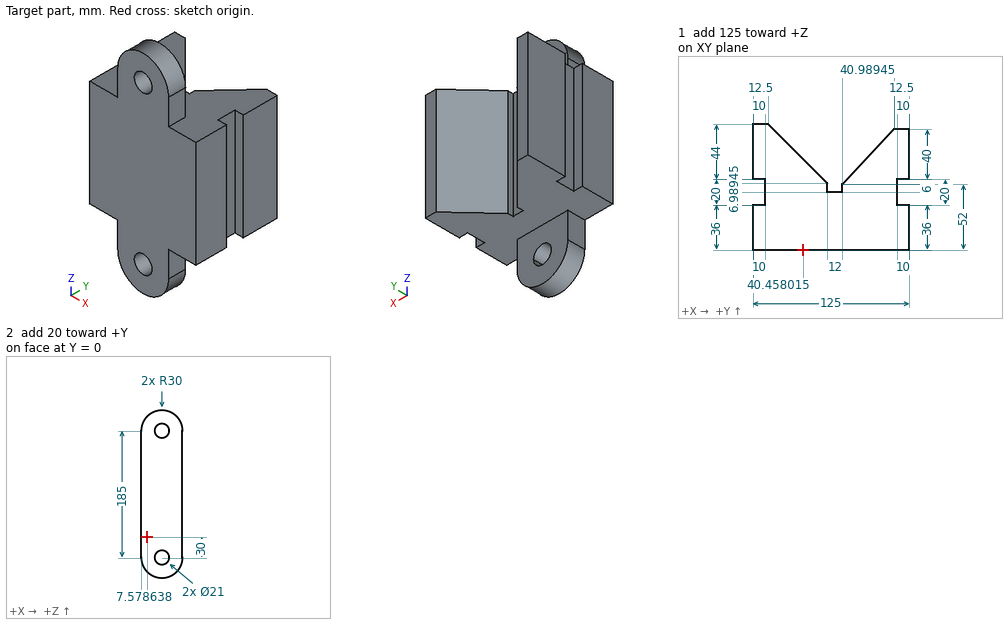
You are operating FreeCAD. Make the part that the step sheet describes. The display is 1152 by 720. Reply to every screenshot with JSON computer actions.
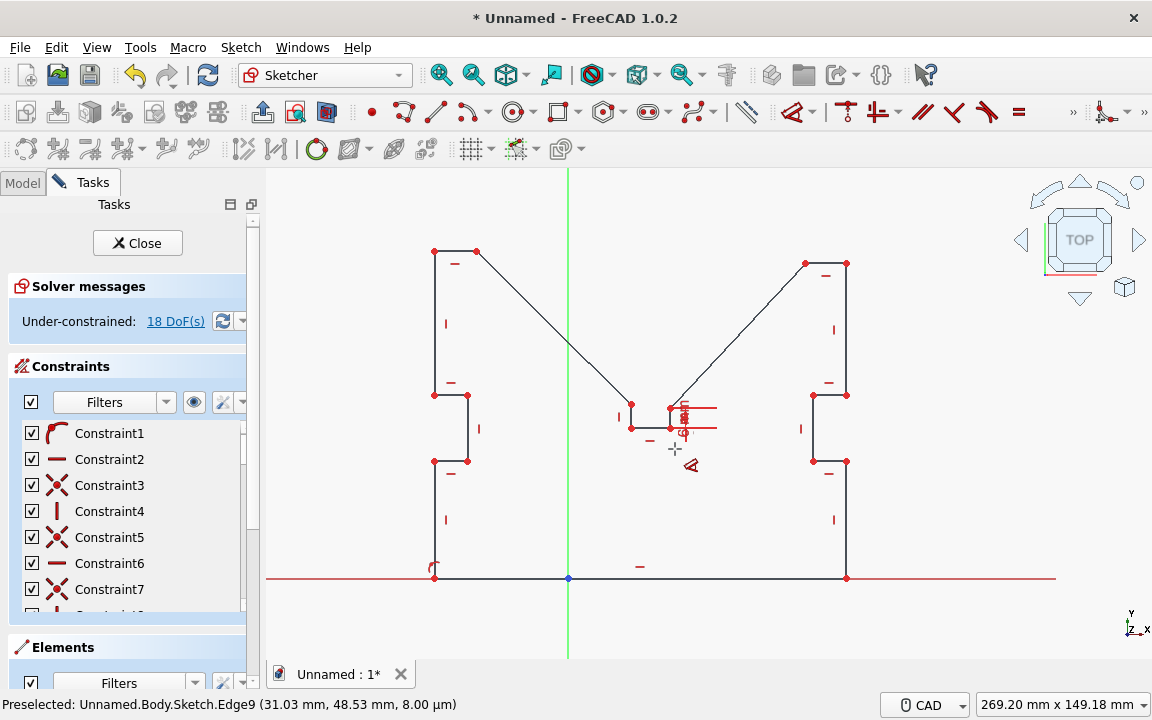
{"action": "left_click", "coordinate": [846, 543]}
{"action": "left_click", "coordinate": [880, 520]}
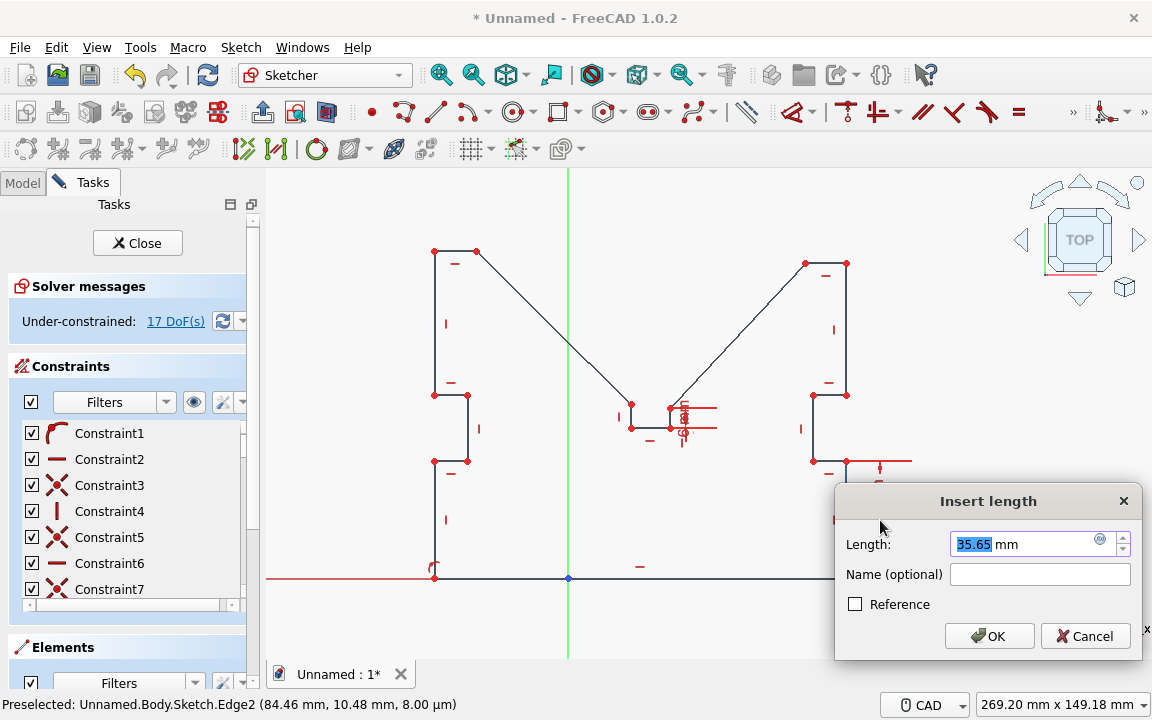
{"action": "type", "text": "36"}
{"action": "key", "text": "Return"}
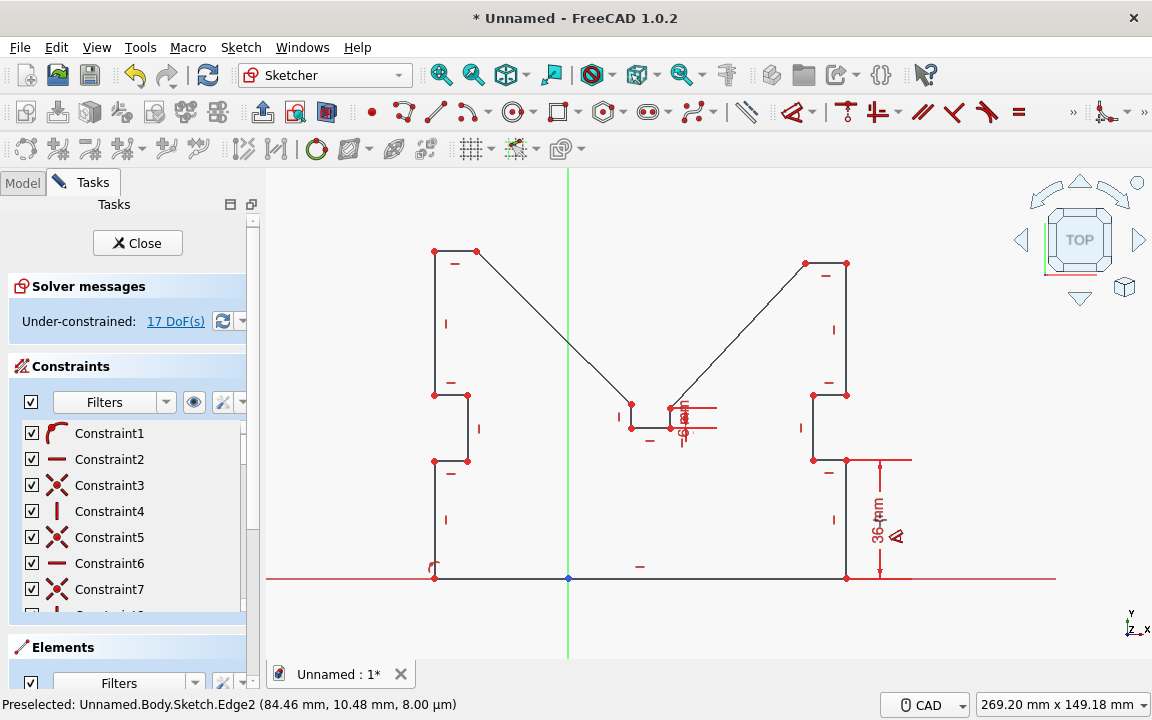
{"action": "scroll", "coordinate": [836, 460], "scroll_direction": "up", "scroll_amount": 2}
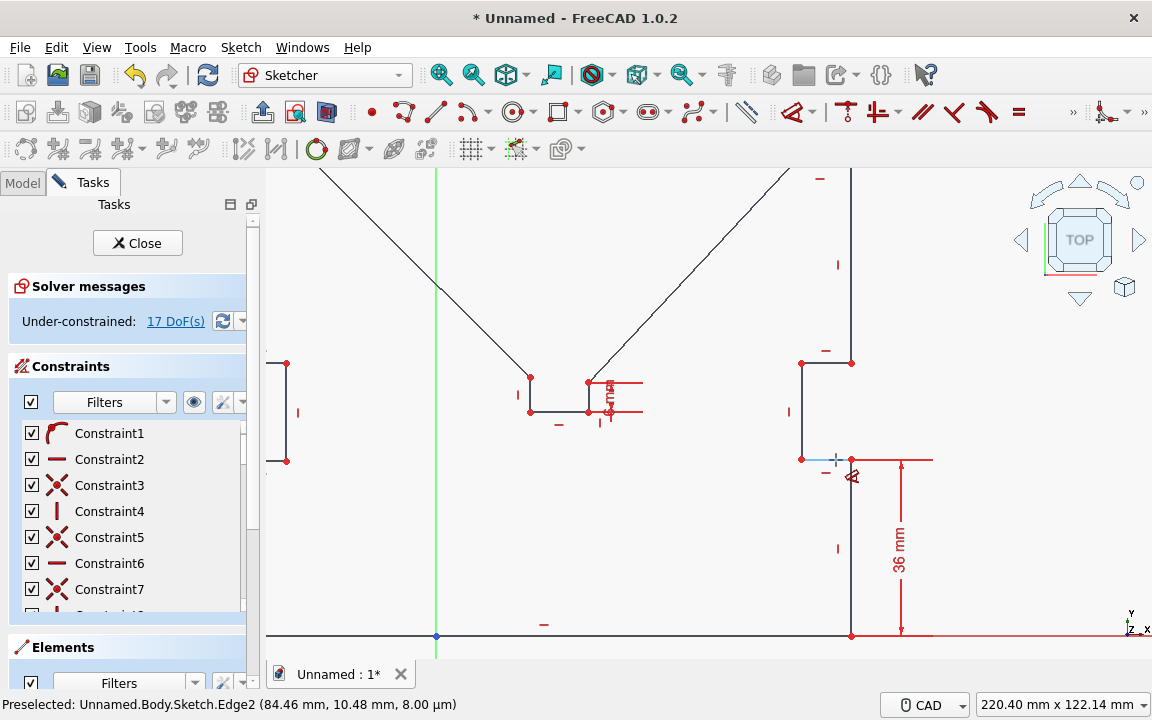
{"action": "left_click", "coordinate": [836, 460]}
{"action": "left_click", "coordinate": [826, 494]}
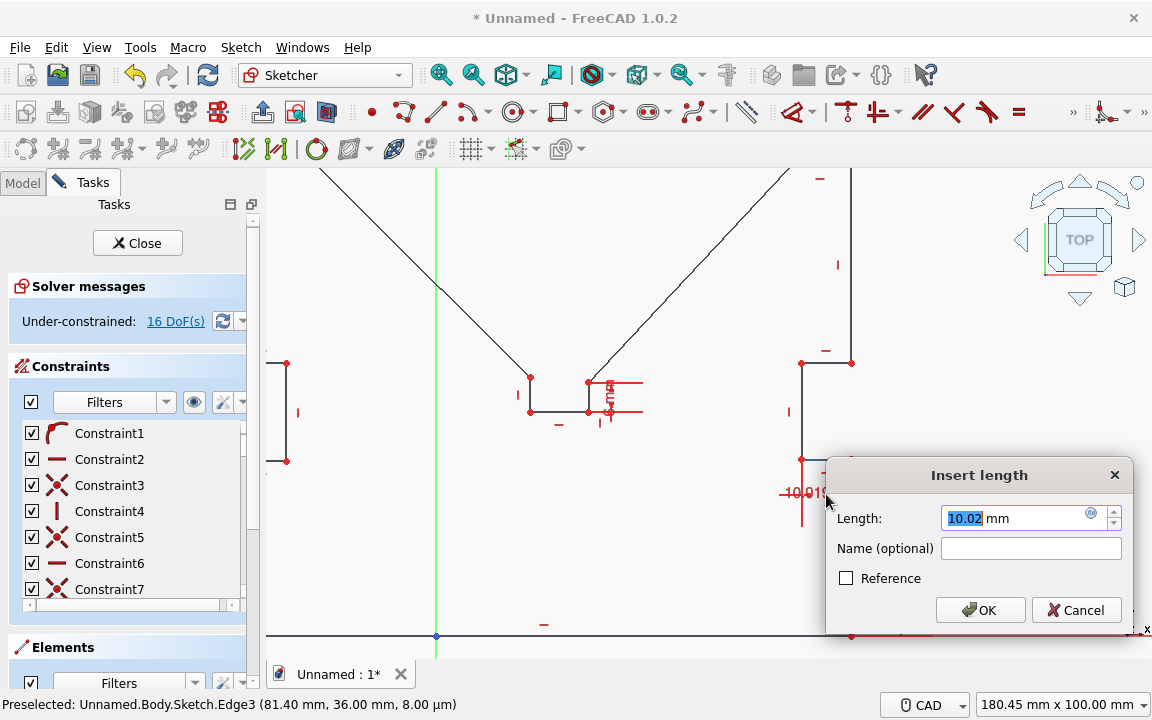
{"action": "type", "text": "10"}
{"action": "key", "text": "Return"}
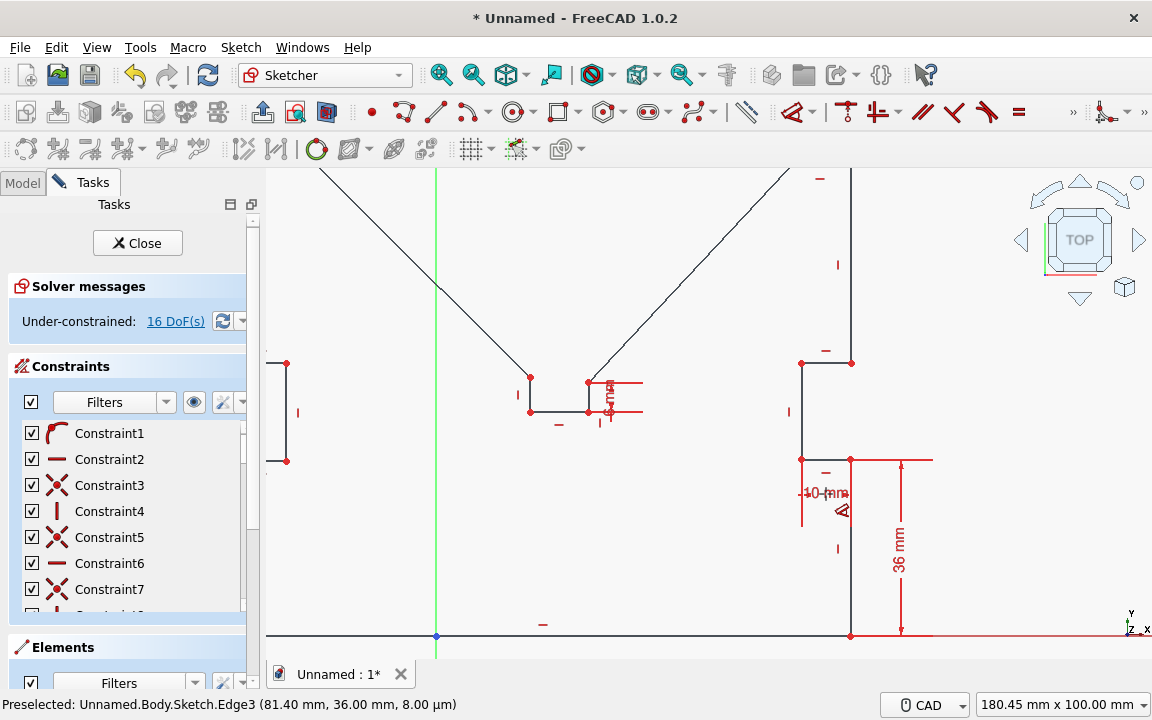
{"action": "left_click", "coordinate": [802, 431]}
{"action": "left_click", "coordinate": [836, 411]}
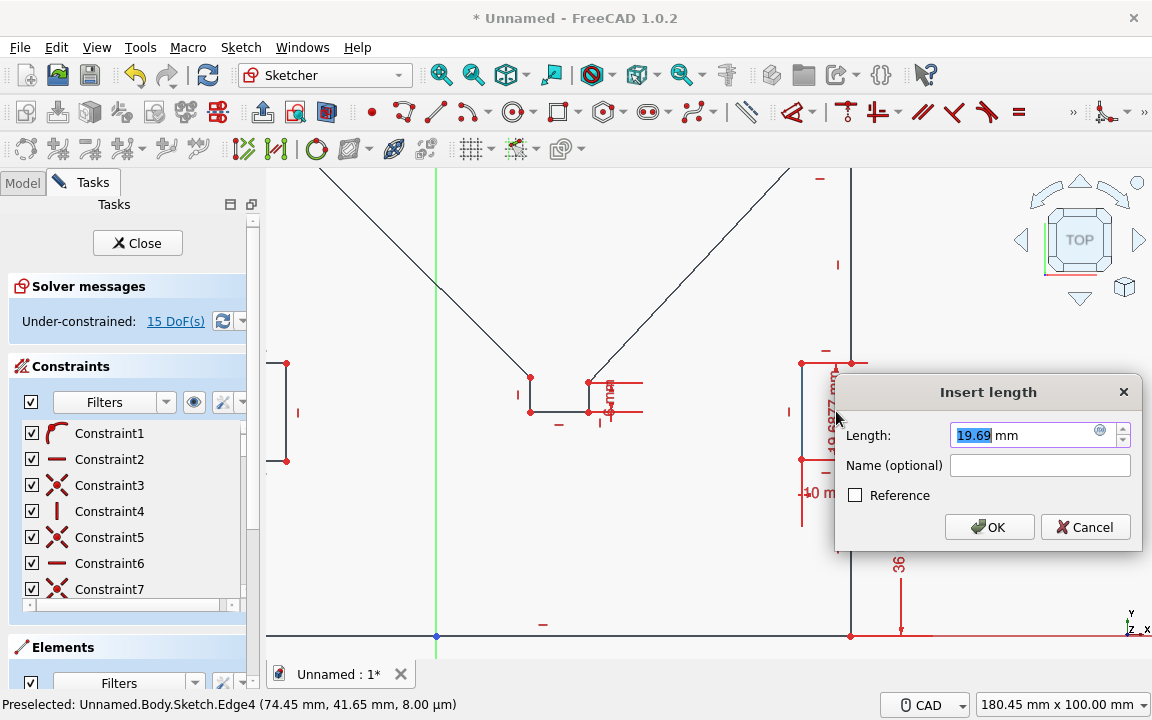
{"action": "type", "text": "20"}
{"action": "key", "text": "Return"}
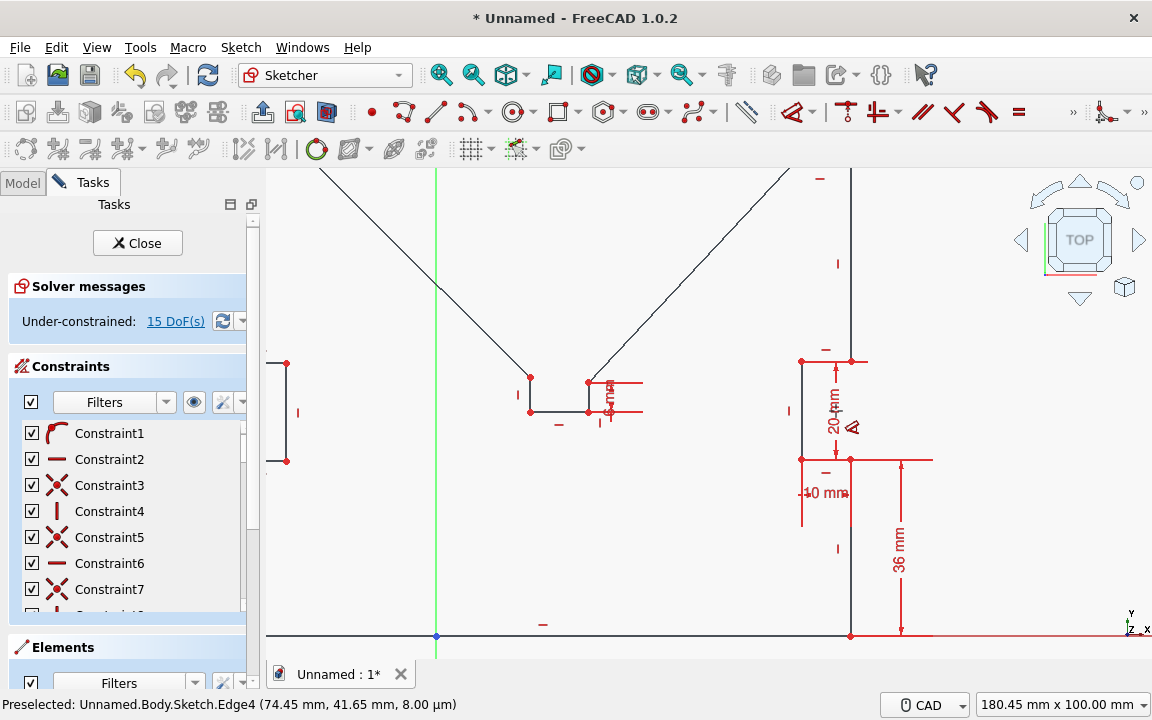
{"action": "left_click", "coordinate": [817, 362]}
{"action": "left_click", "coordinate": [826, 328]}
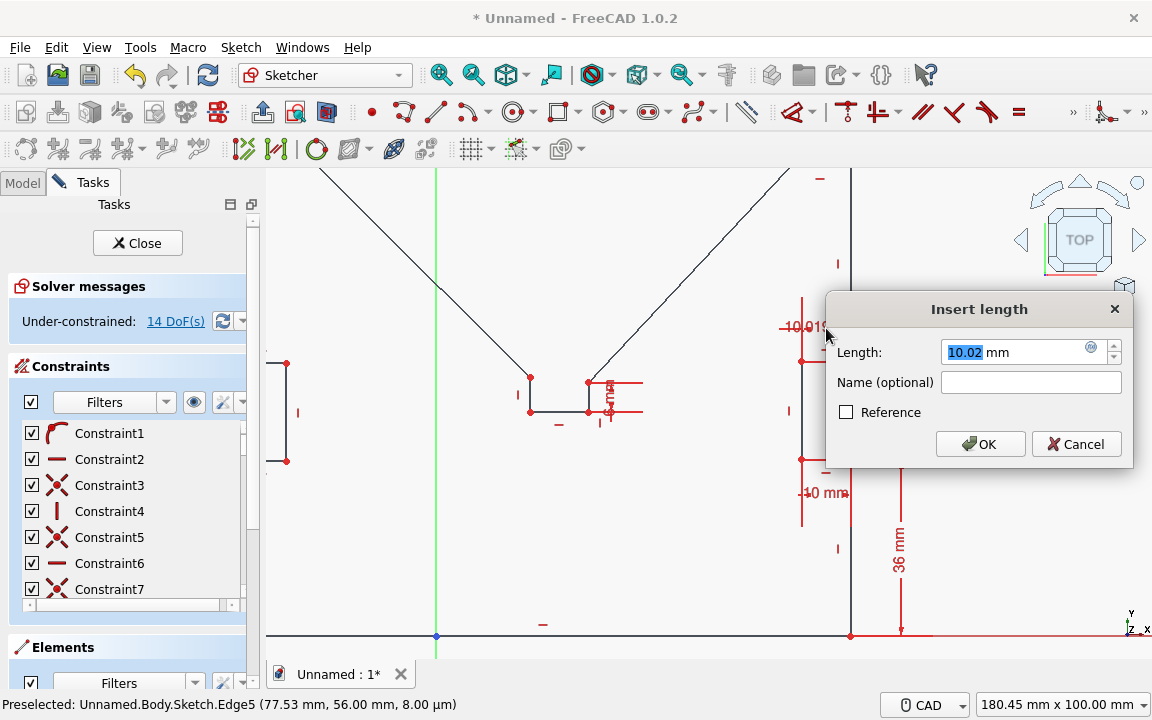
{"action": "type", "text": "10"}
{"action": "key", "text": "Return"}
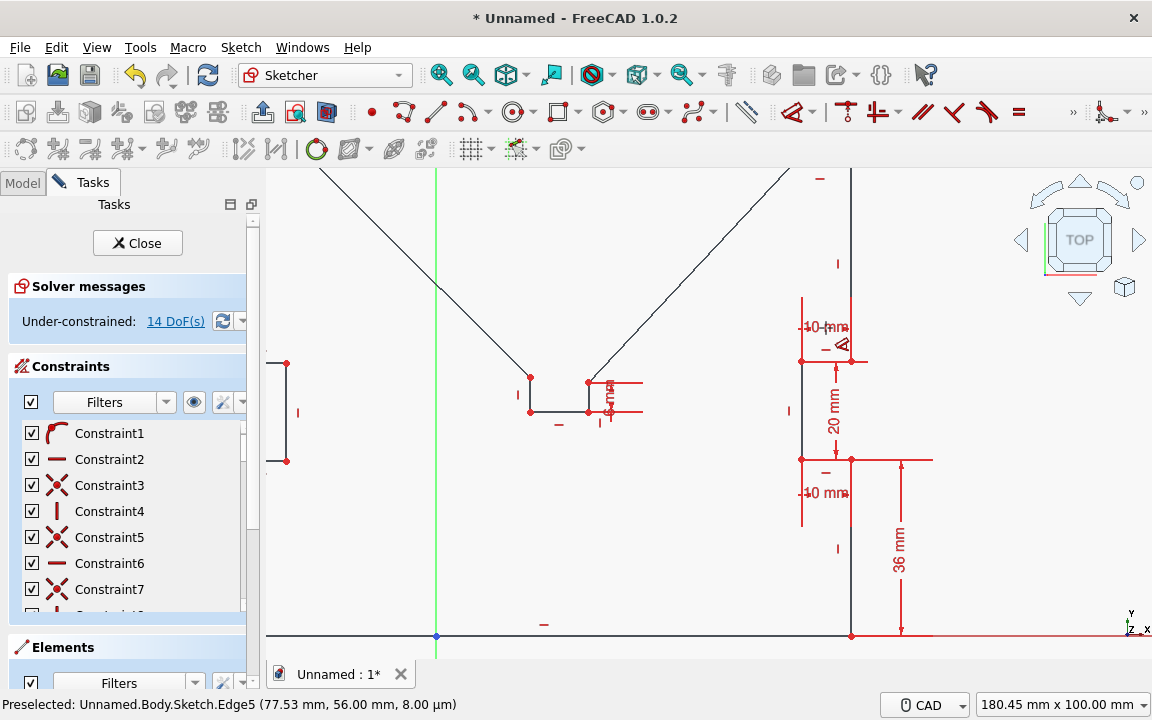
{"action": "left_click", "coordinate": [851, 303]}
{"action": "left_click", "coordinate": [885, 279]}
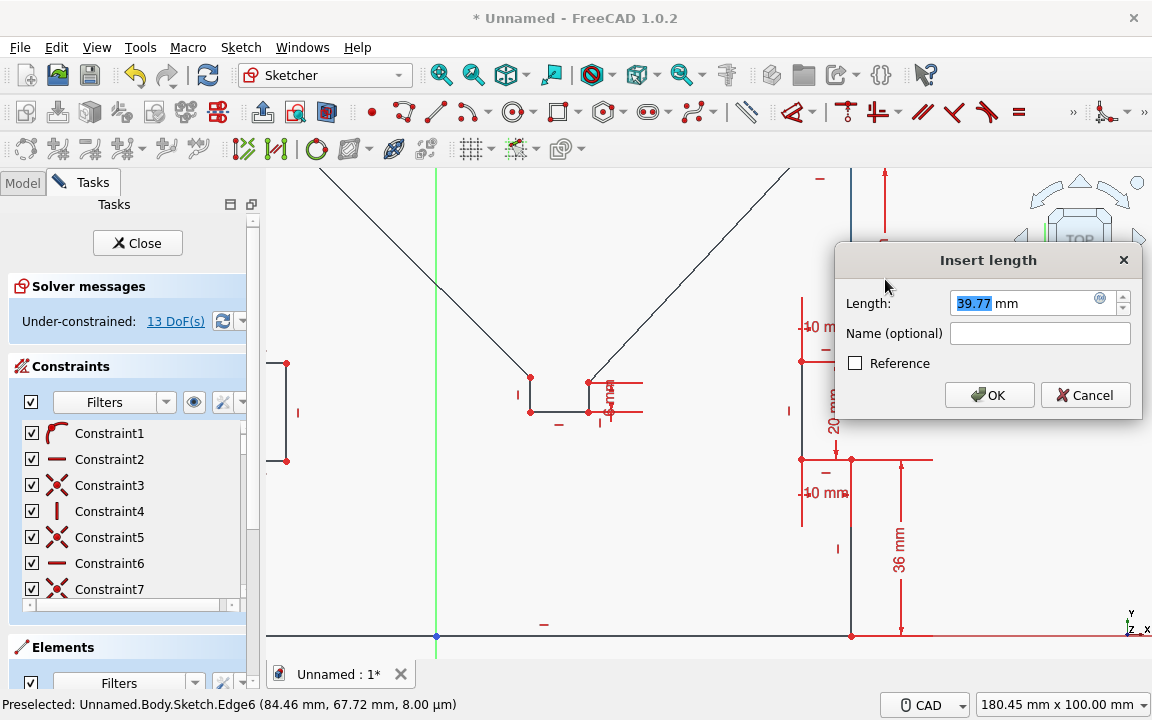
{"action": "type", "text": "40"}
{"action": "key", "text": "Return"}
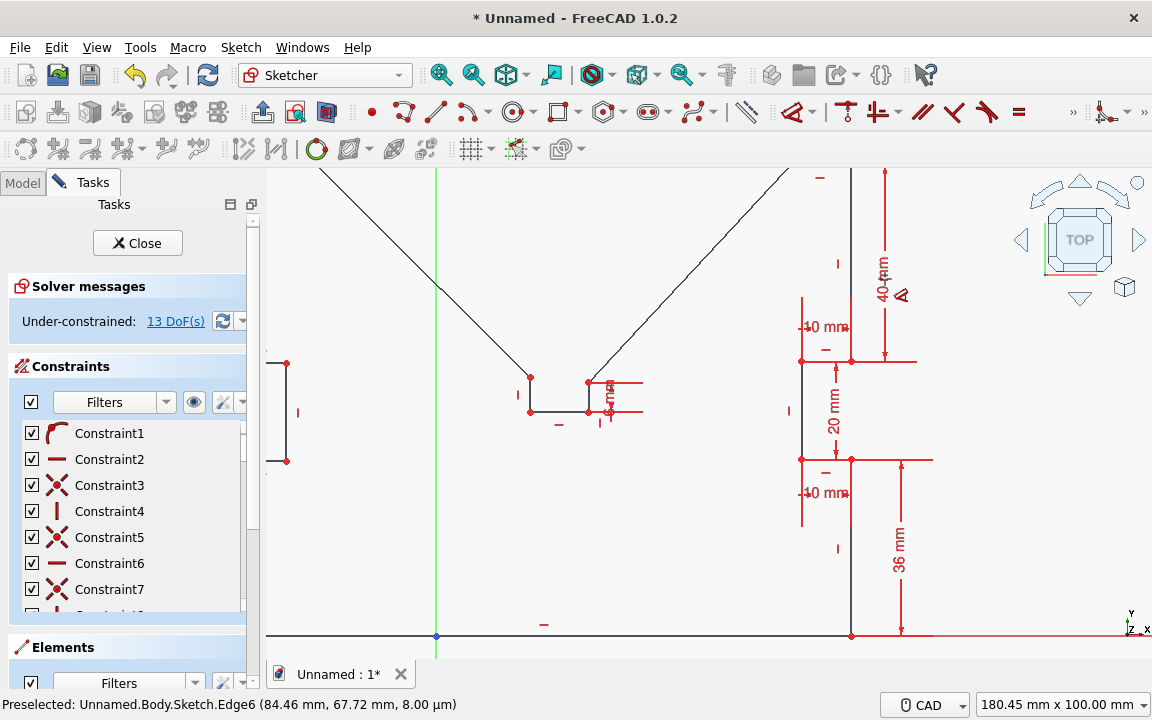
{"action": "left_click", "coordinate": [571, 412]}
{"action": "left_click", "coordinate": [560, 446]}